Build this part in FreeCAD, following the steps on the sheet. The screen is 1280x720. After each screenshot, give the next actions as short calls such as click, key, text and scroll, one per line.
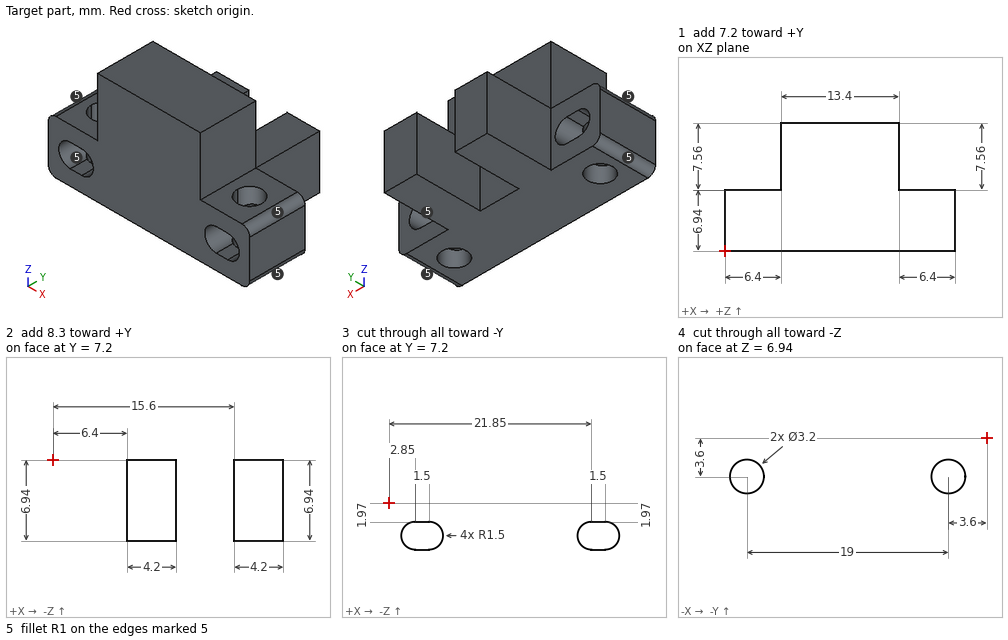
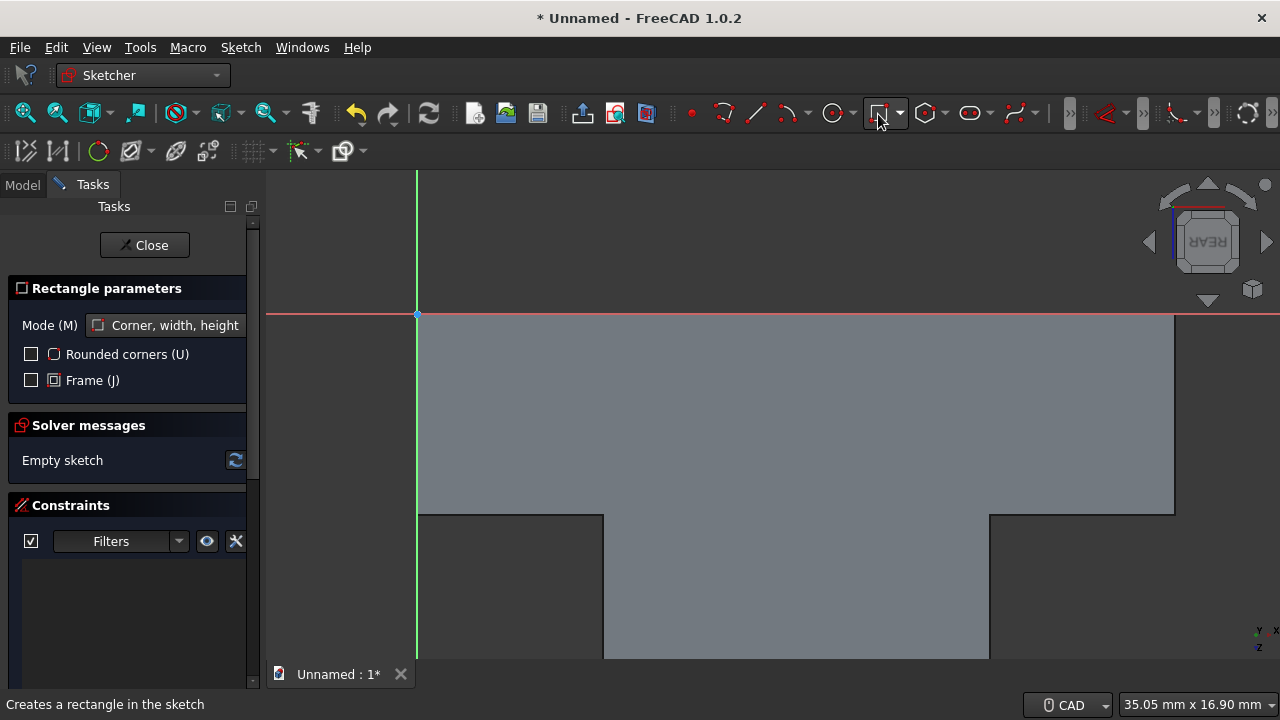
click(603, 314)
click(724, 515)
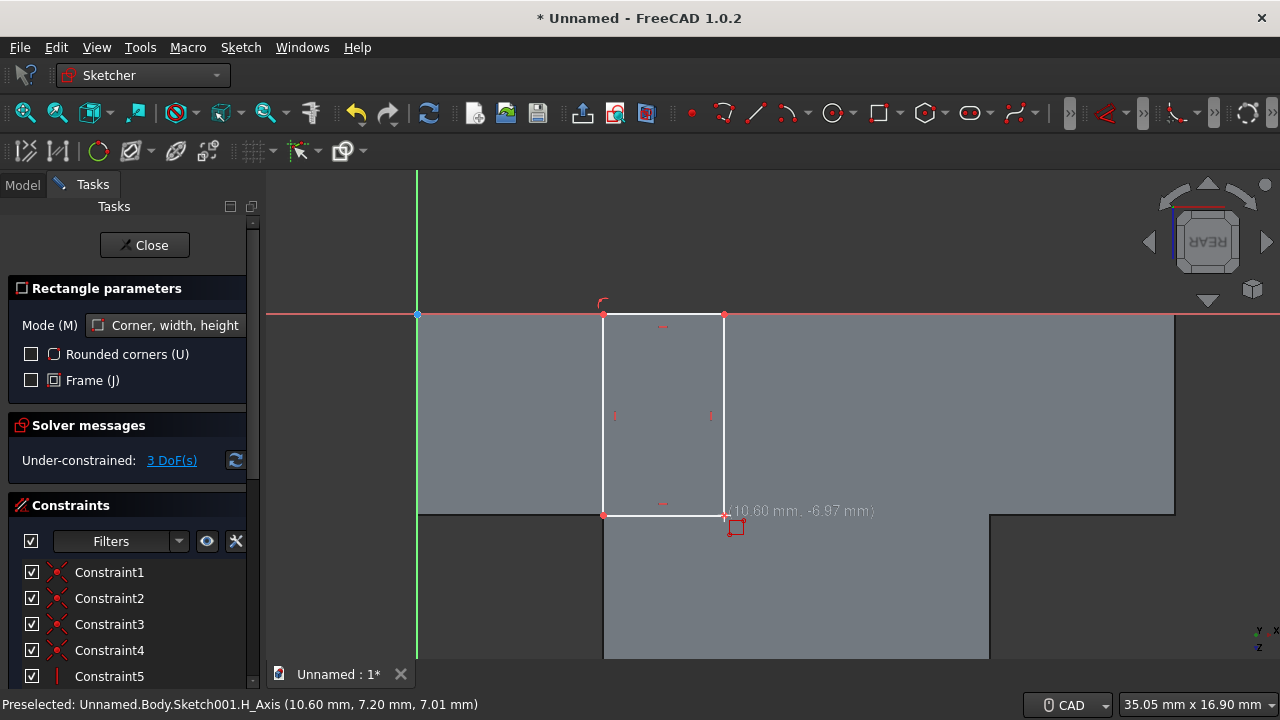
click(869, 314)
click(990, 515)
key(Escape)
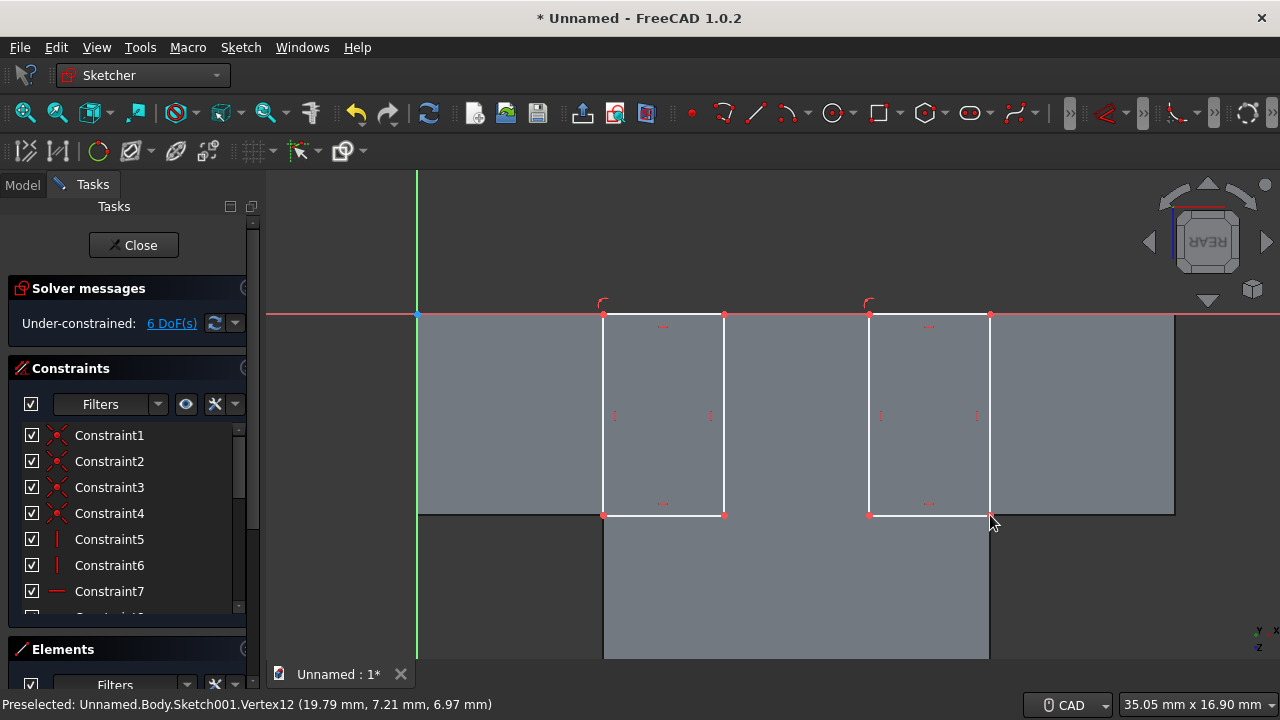
click(1106, 114)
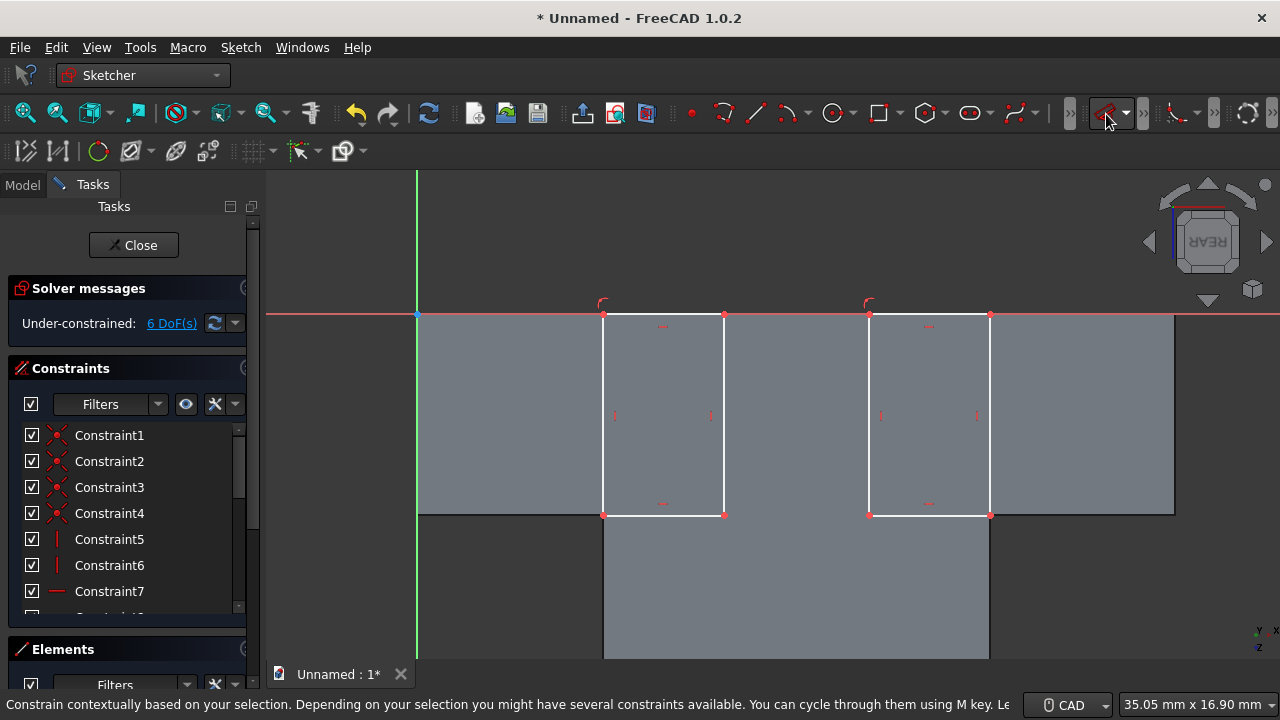
click(639, 516)
click(664, 550)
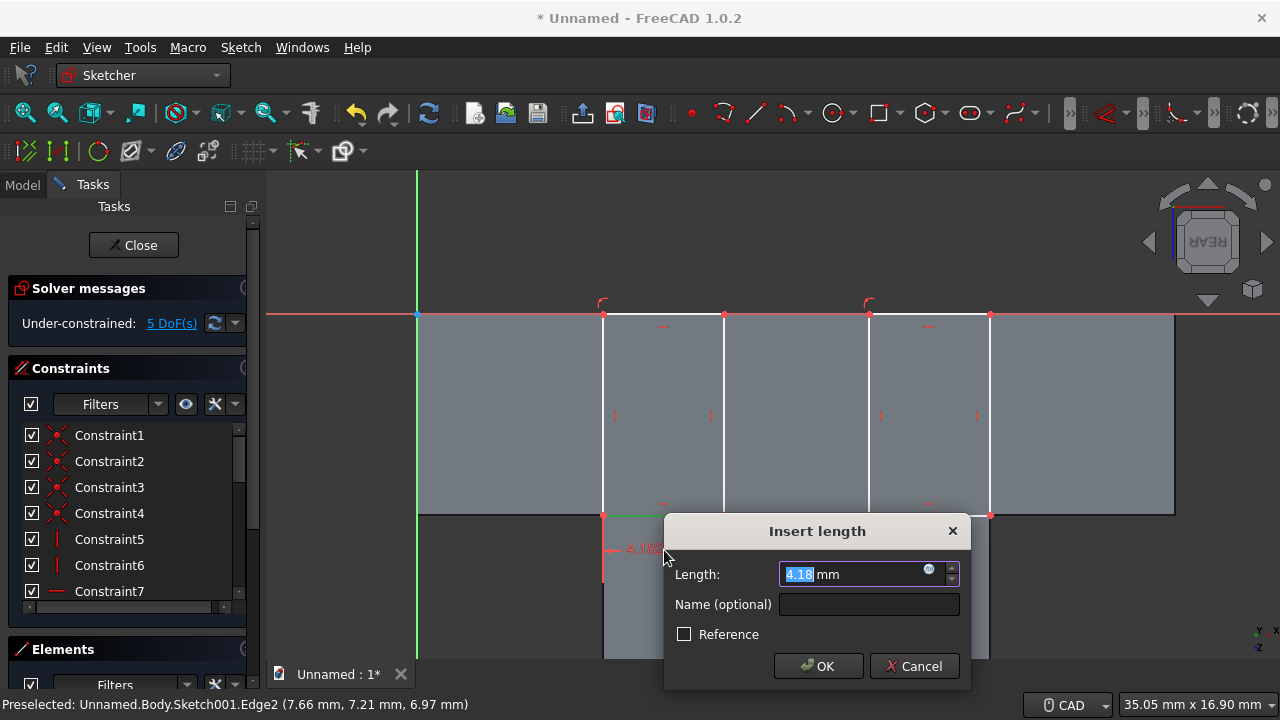
text(4.2)
key(Return)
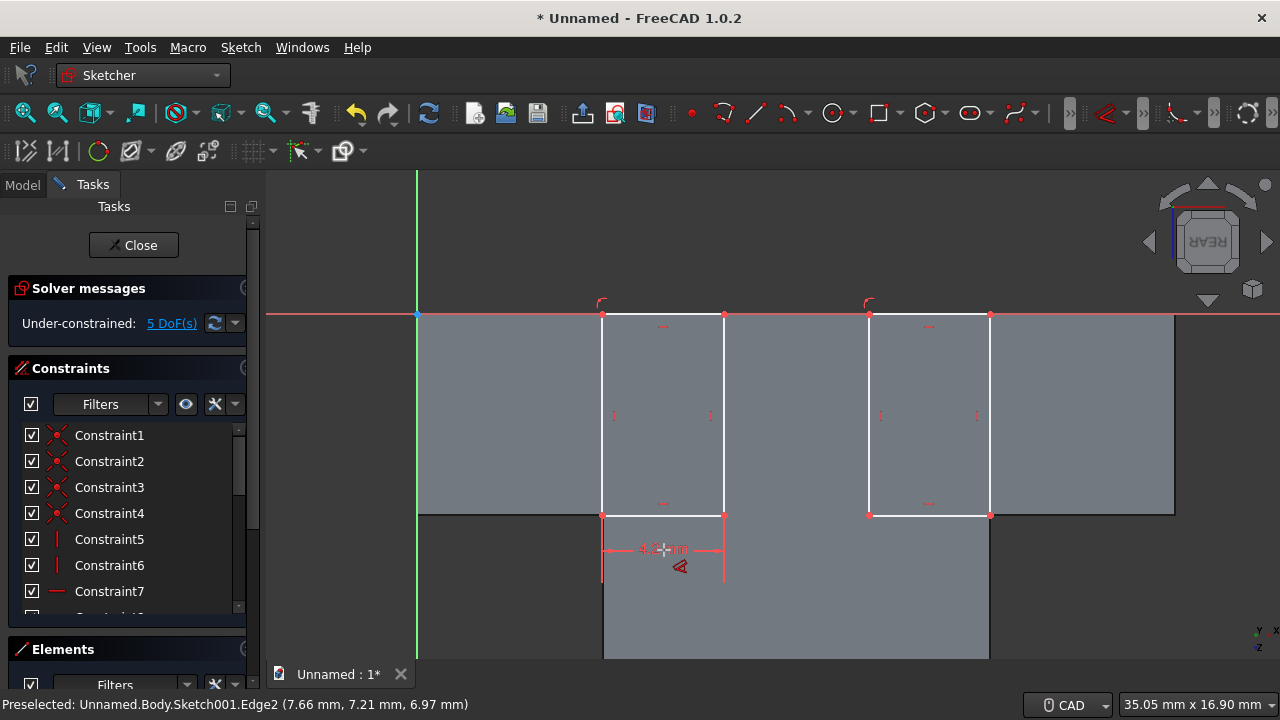
click(905, 516)
click(929, 550)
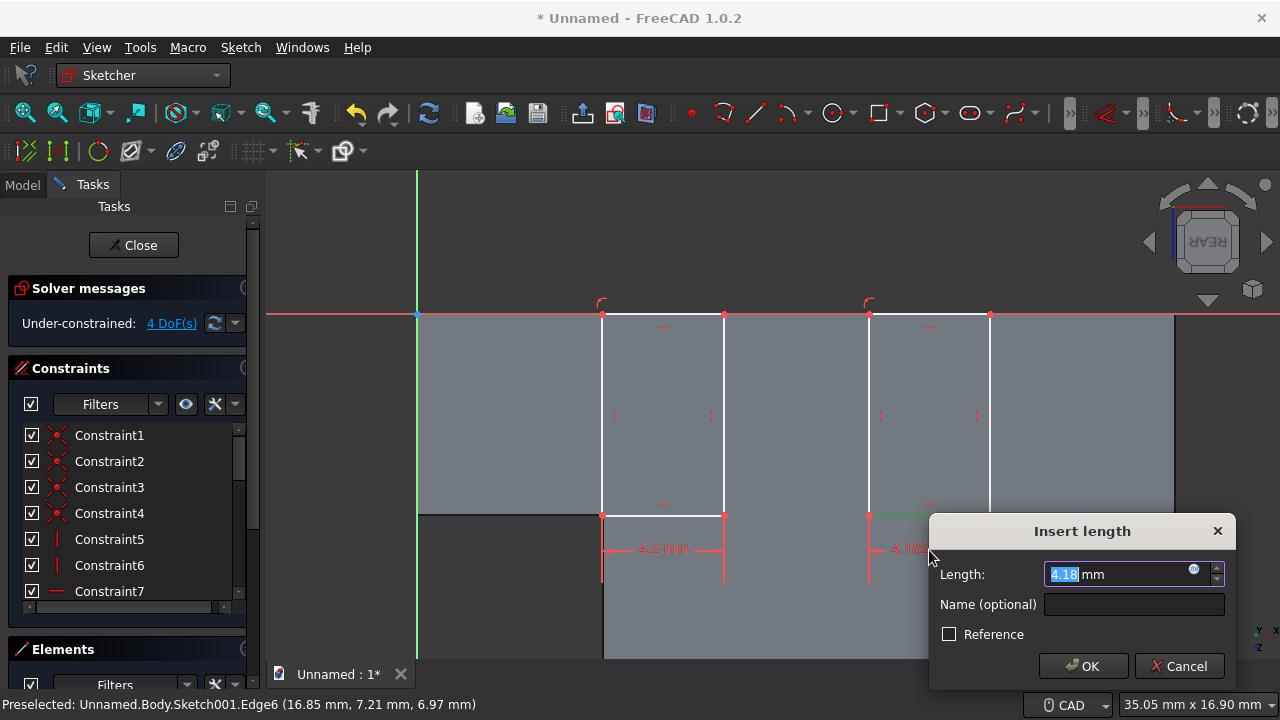
text(4.2)
key(Return)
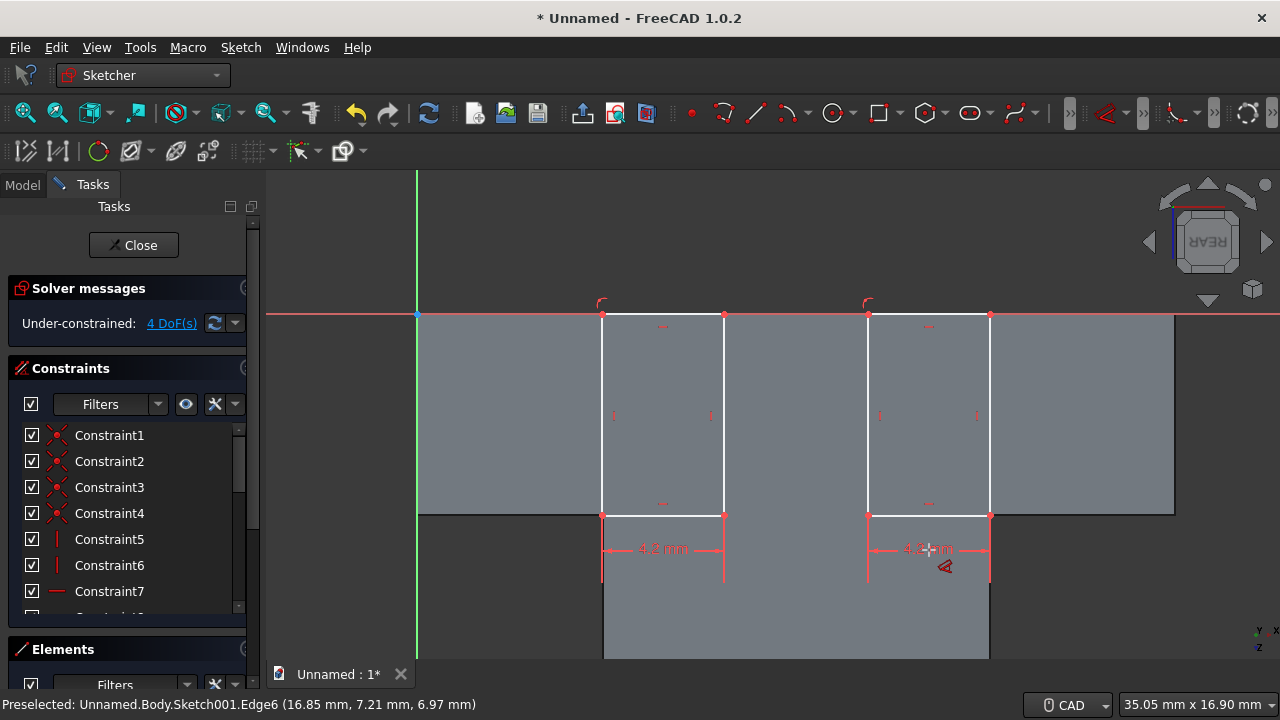
click(602, 375)
click(568, 415)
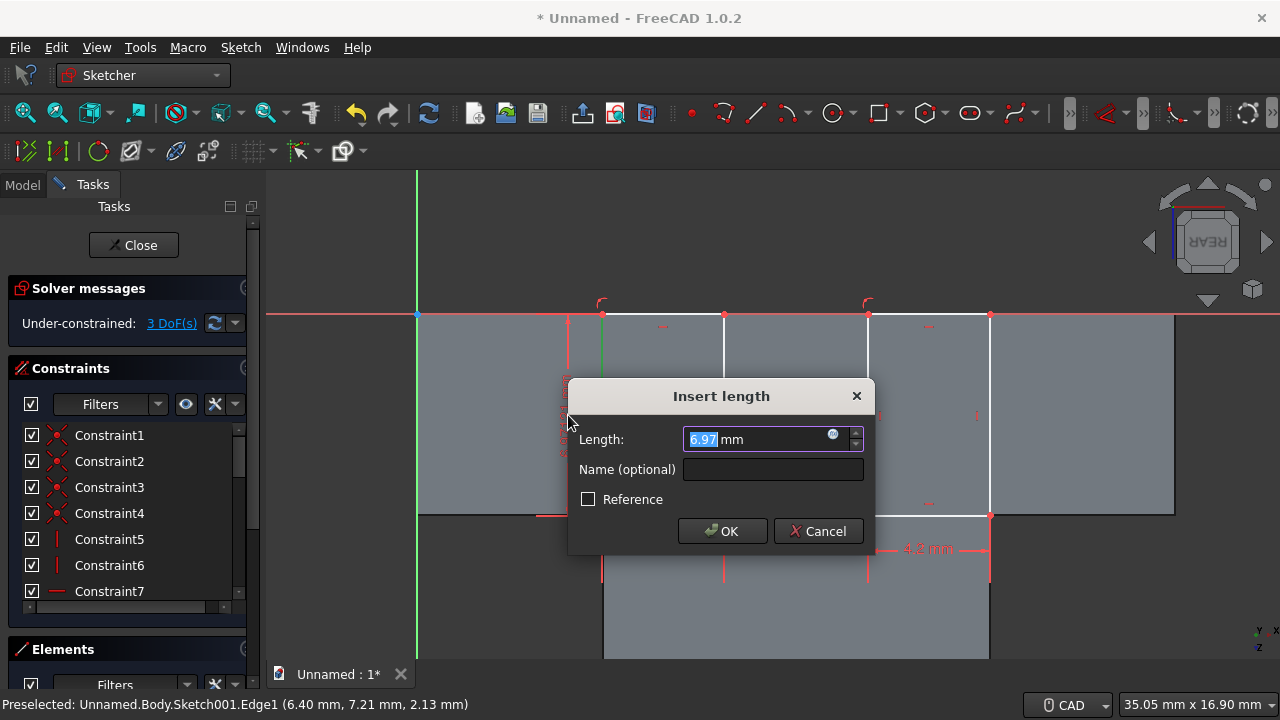
text(6.94)
key(Return)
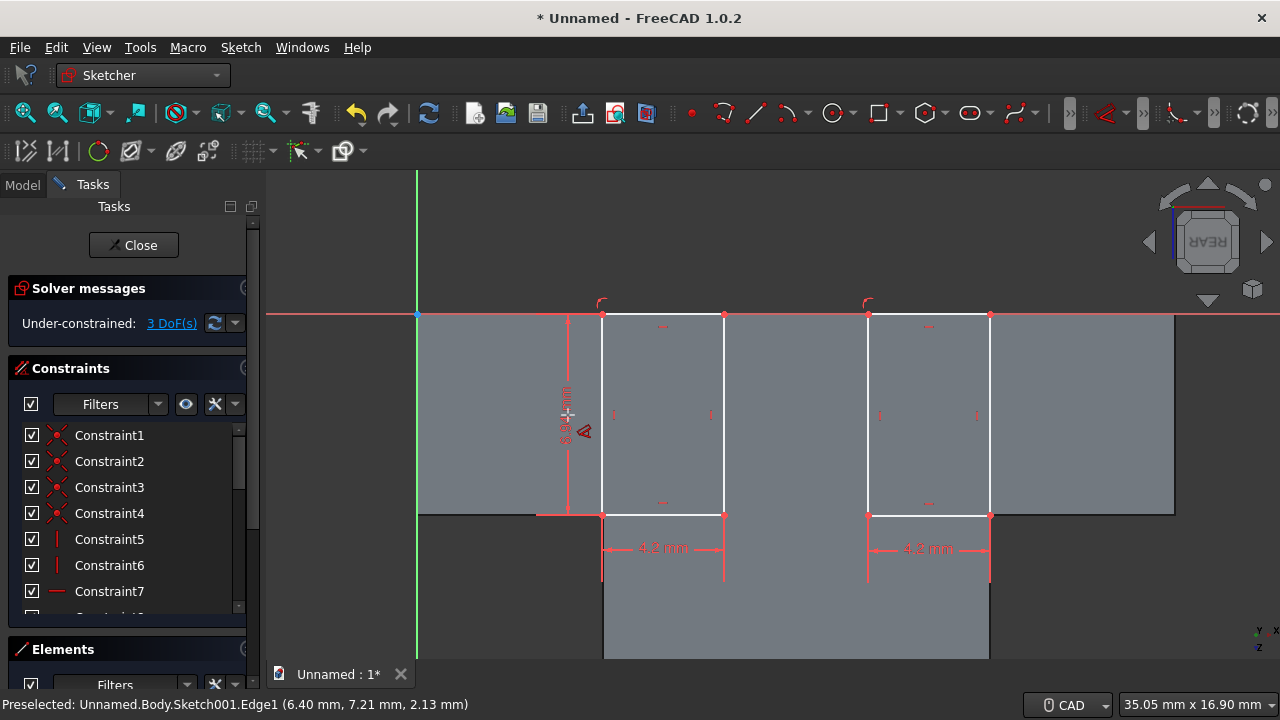
click(868, 375)
click(902, 415)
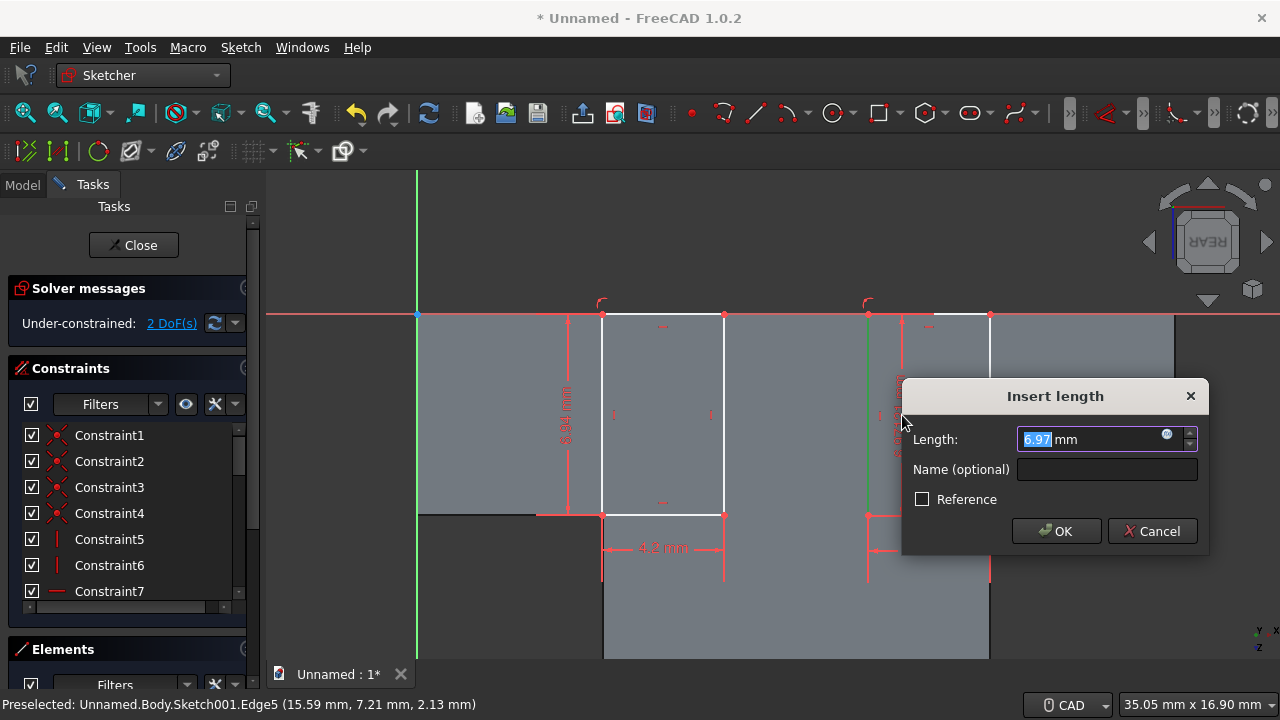
text(6.94)
key(Return)